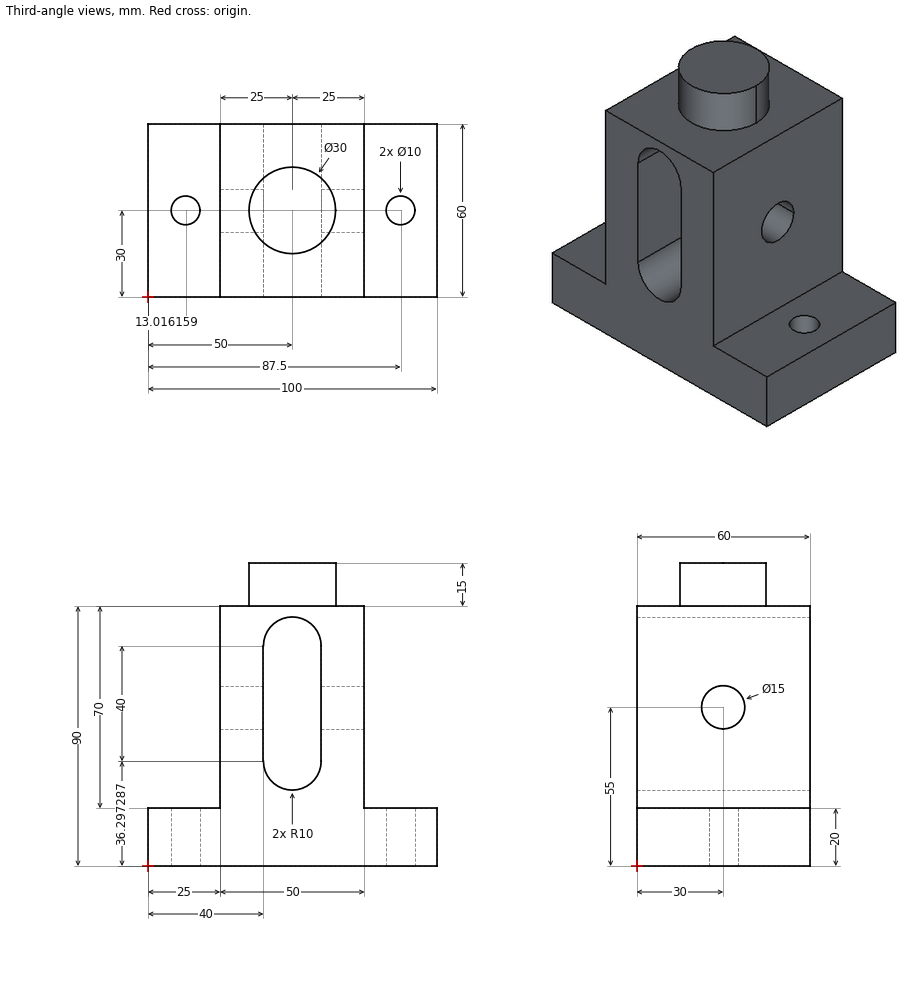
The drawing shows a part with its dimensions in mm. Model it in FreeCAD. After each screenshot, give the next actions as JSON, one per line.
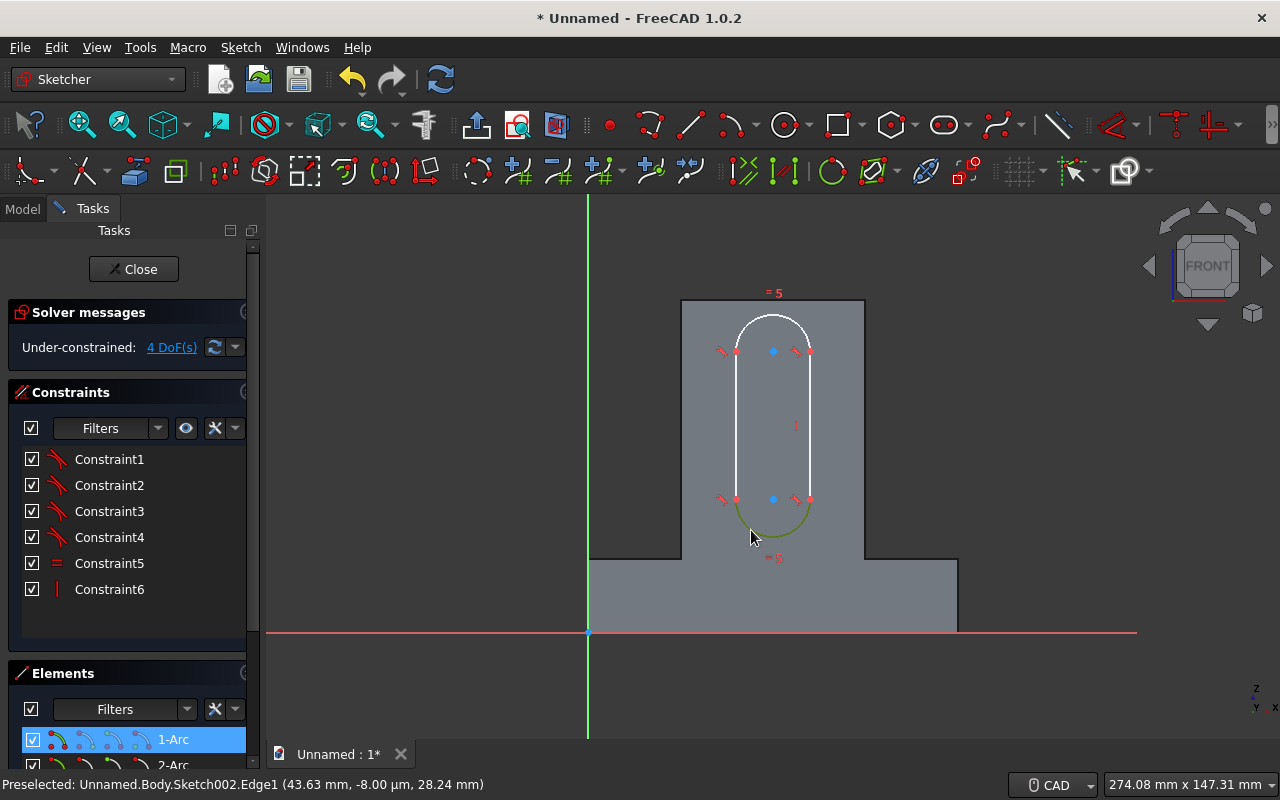
{"action": "key", "text": "k r"}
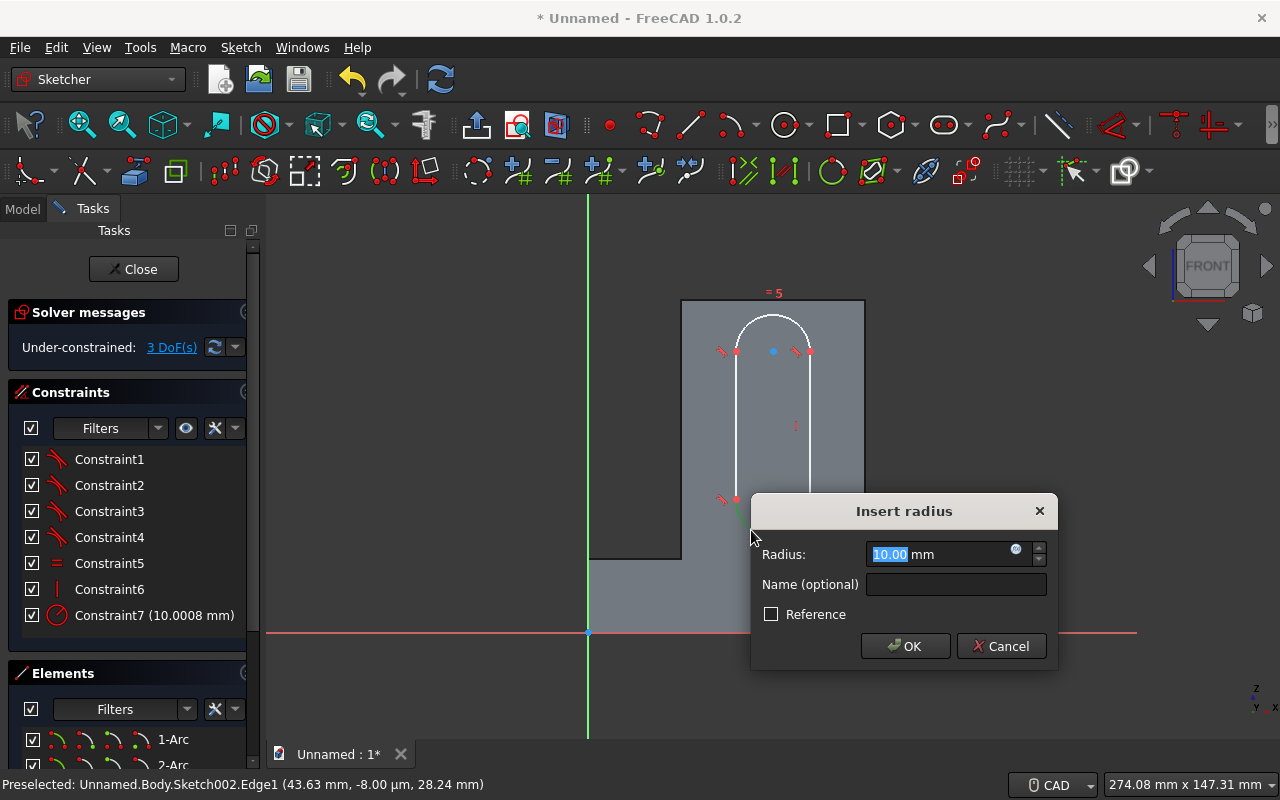
{"action": "type", "text": "10"}
{"action": "key", "text": "Return"}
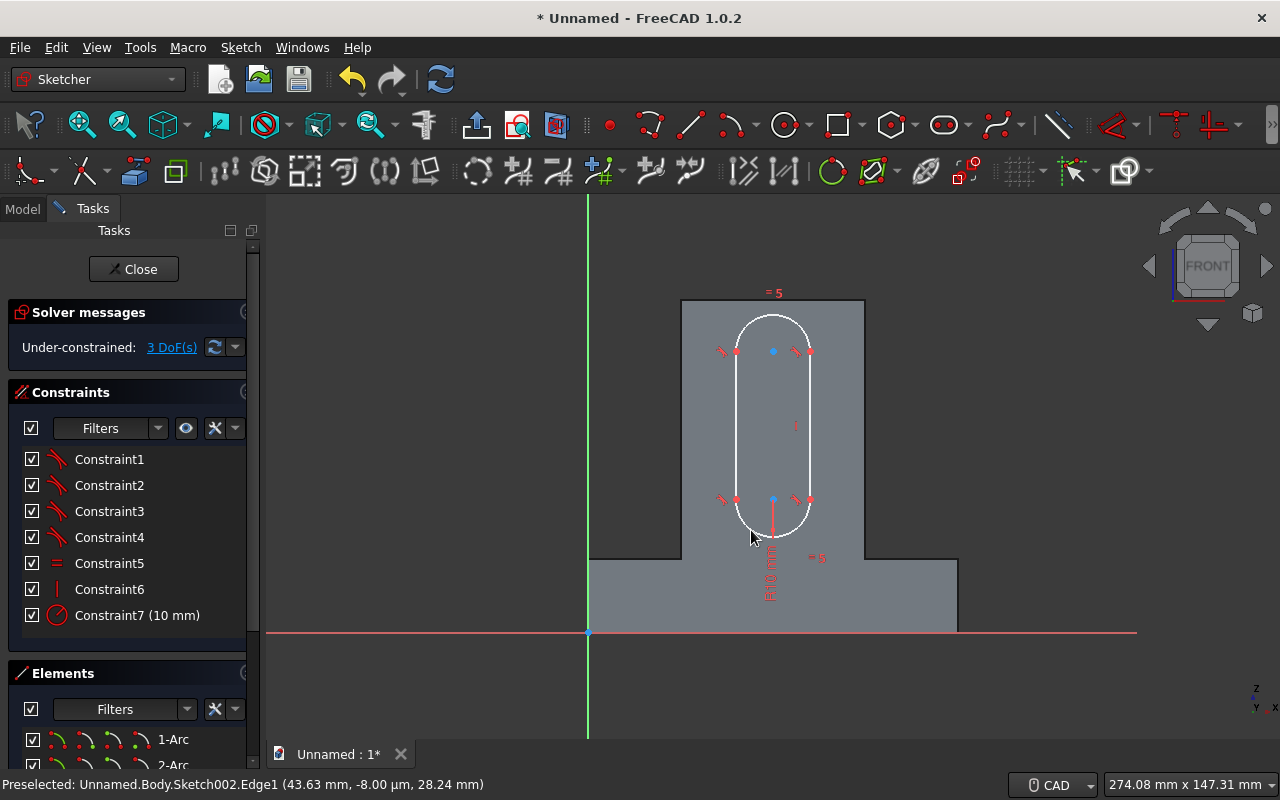
{"action": "left_click", "coordinate": [736, 456]}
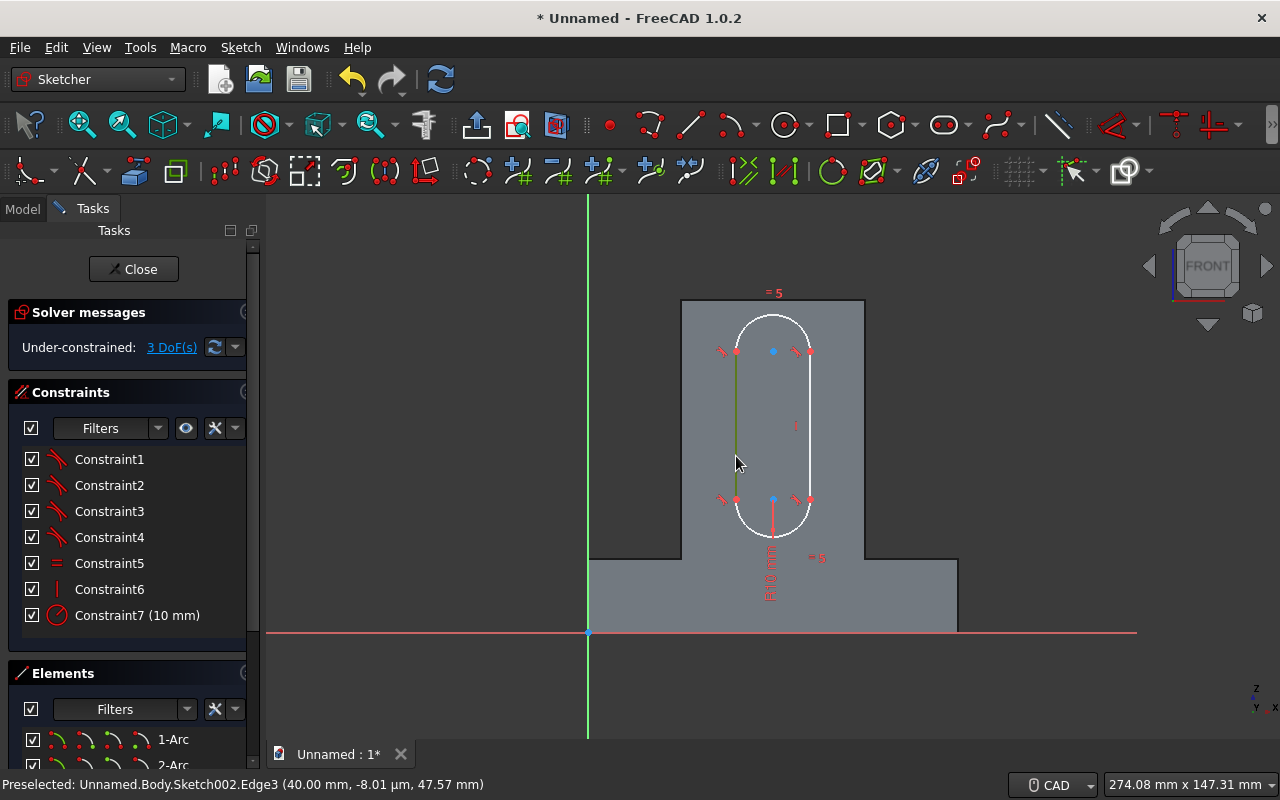
{"action": "key", "text": "i"}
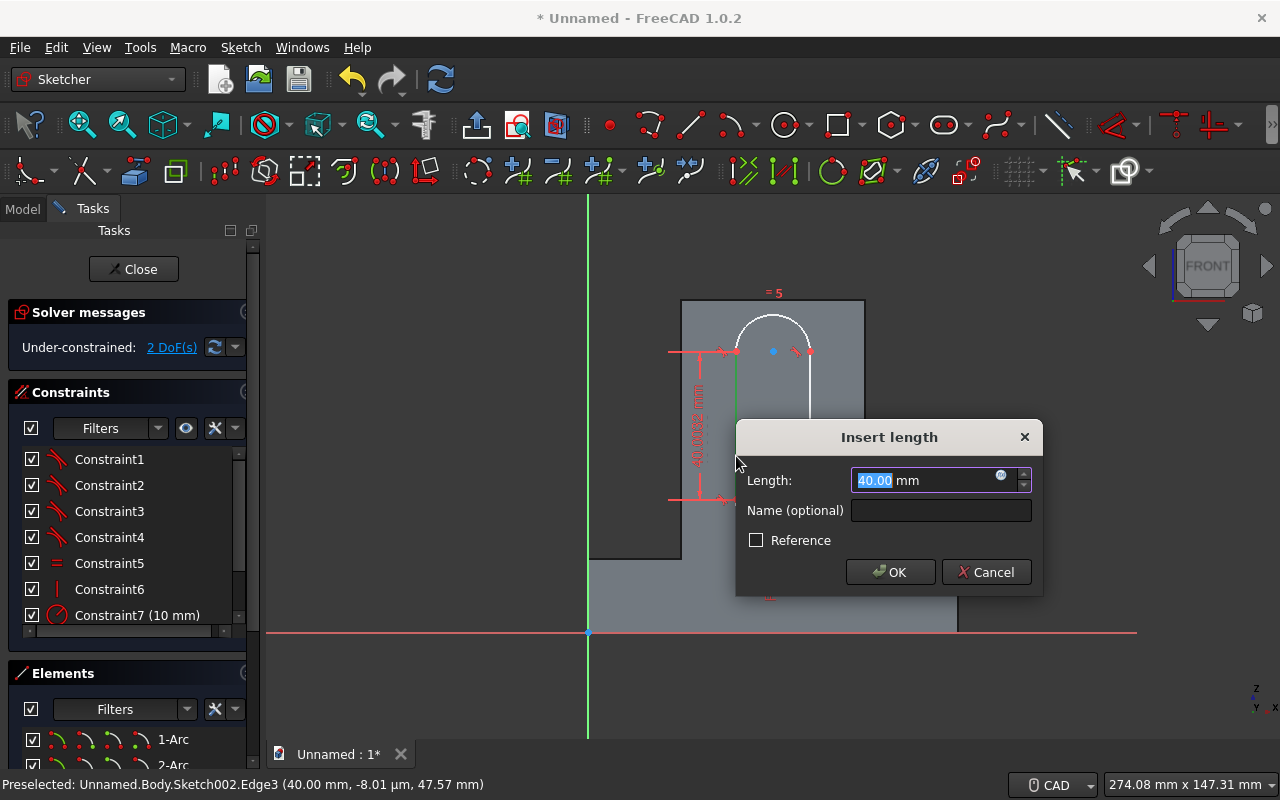
{"action": "type", "text": "40"}
{"action": "key", "text": "Return"}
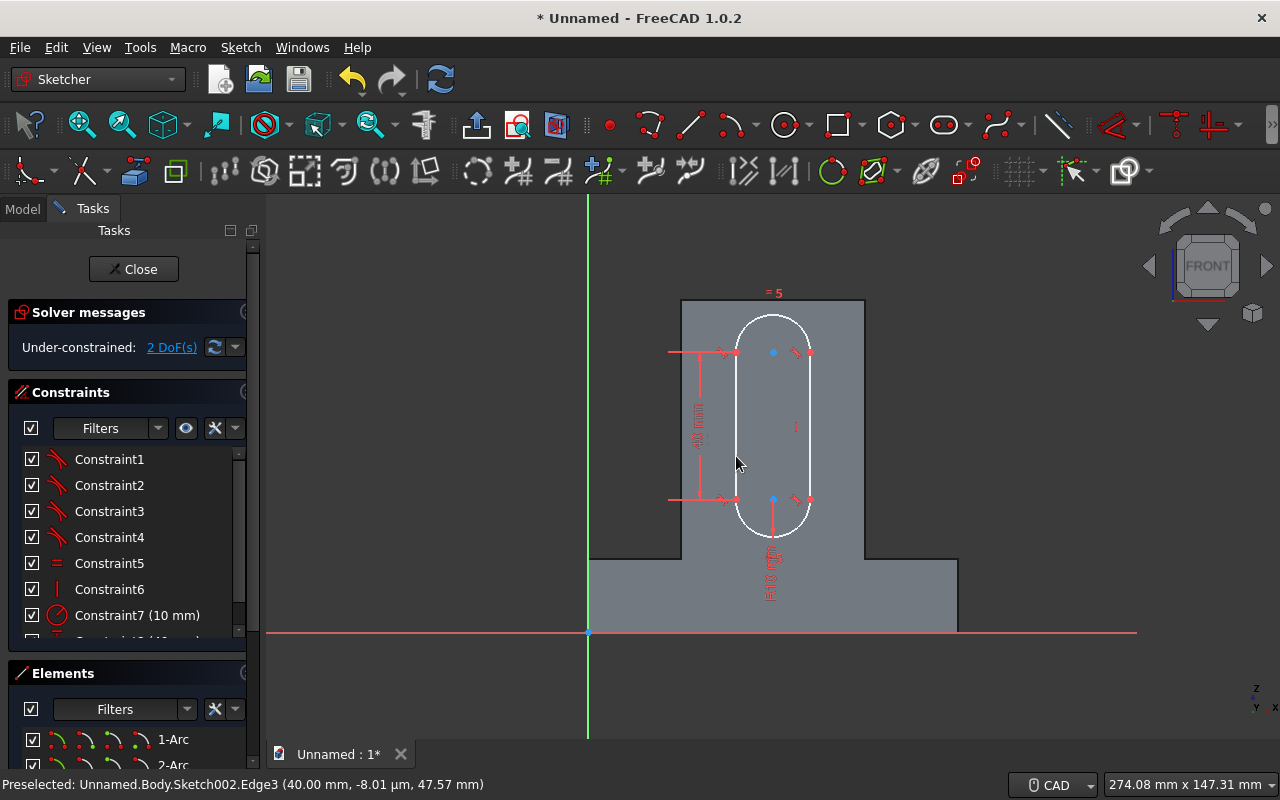
{"action": "left_click", "coordinate": [736, 500]}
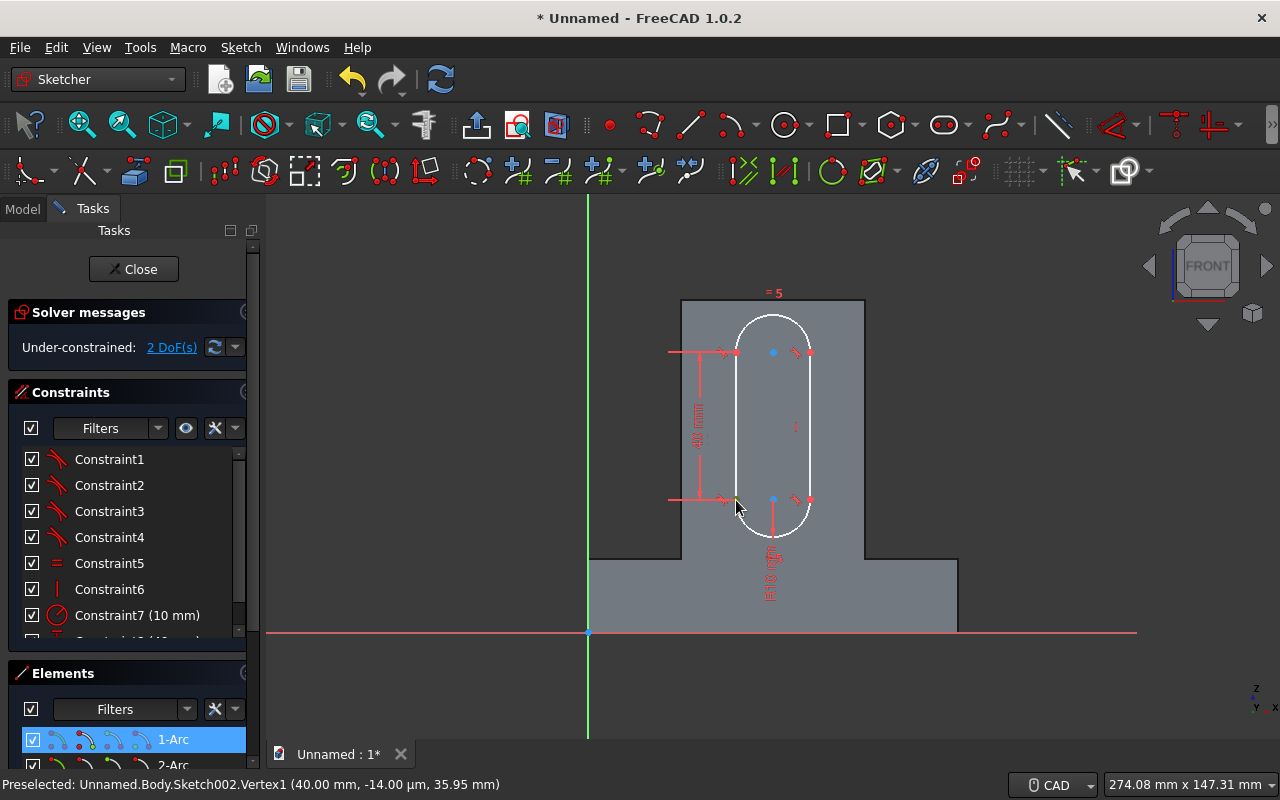
{"action": "left_click", "coordinate": [1138, 126]}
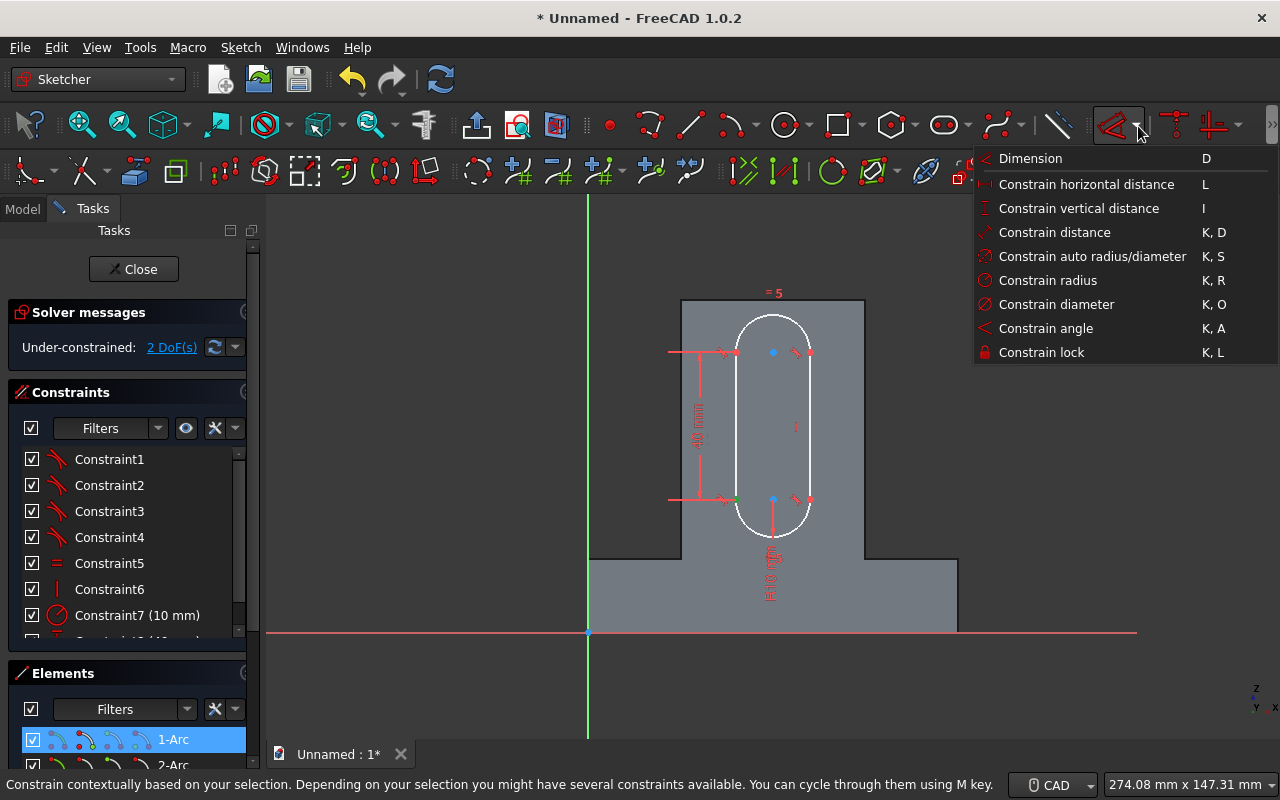
{"action": "left_click", "coordinate": [1126, 184]}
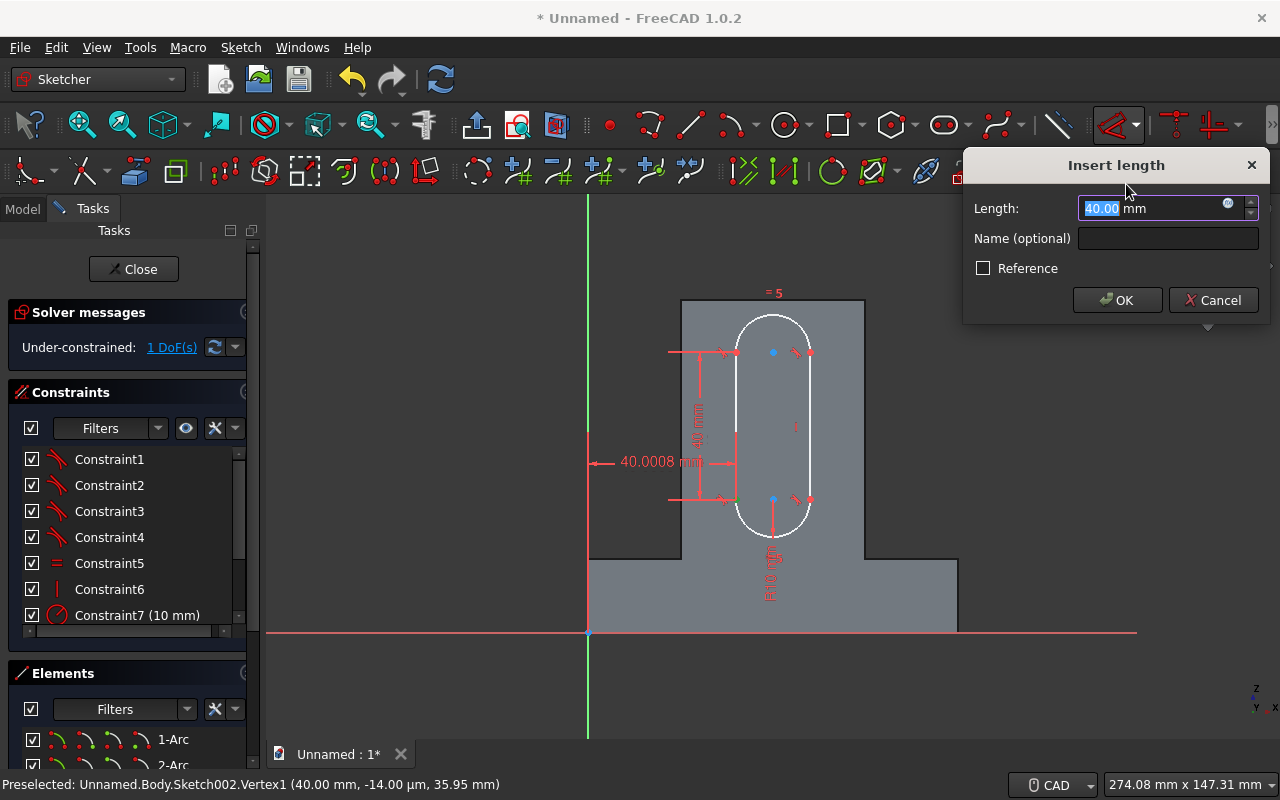
{"action": "type", "text": "40"}
{"action": "key", "text": "Return"}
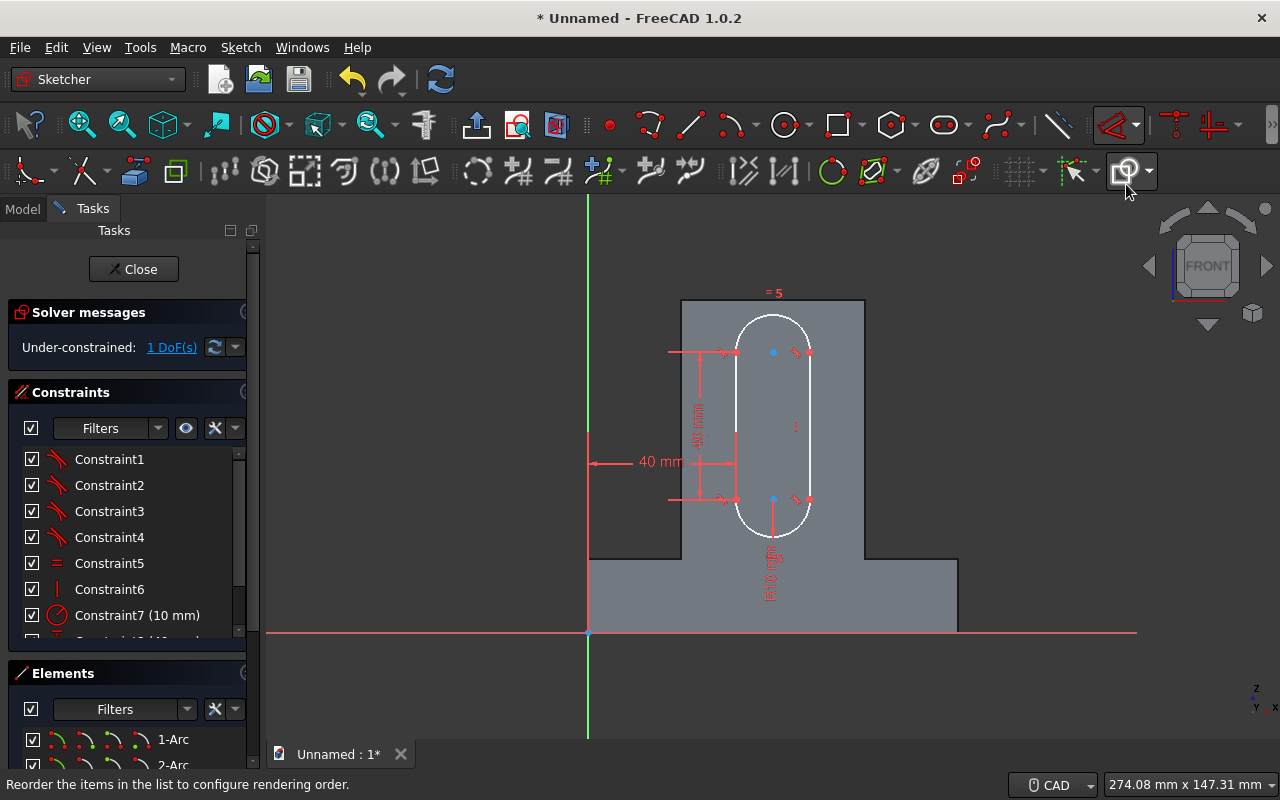
{"action": "left_click", "coordinate": [736, 500]}